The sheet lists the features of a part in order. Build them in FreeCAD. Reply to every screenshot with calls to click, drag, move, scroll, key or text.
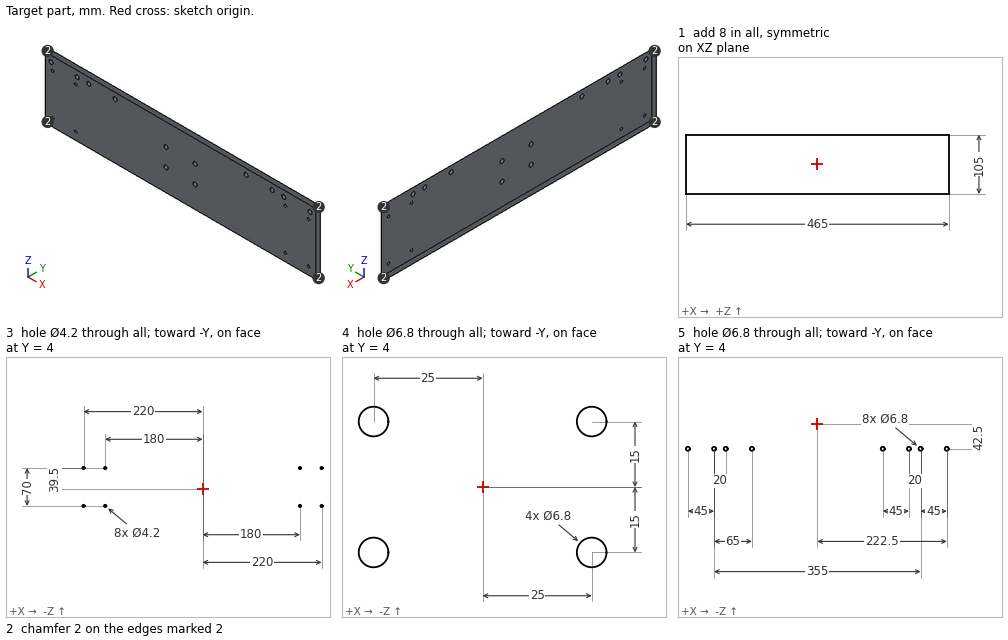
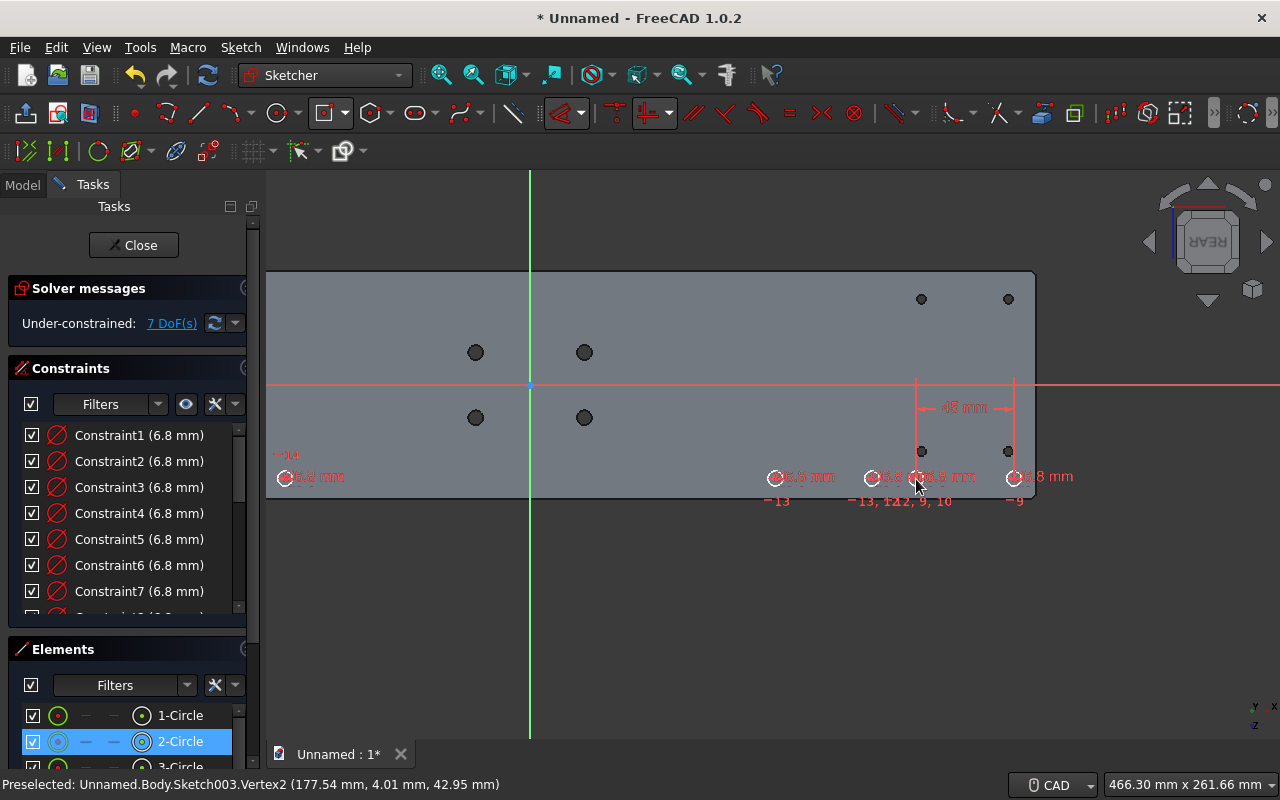
click(872, 479)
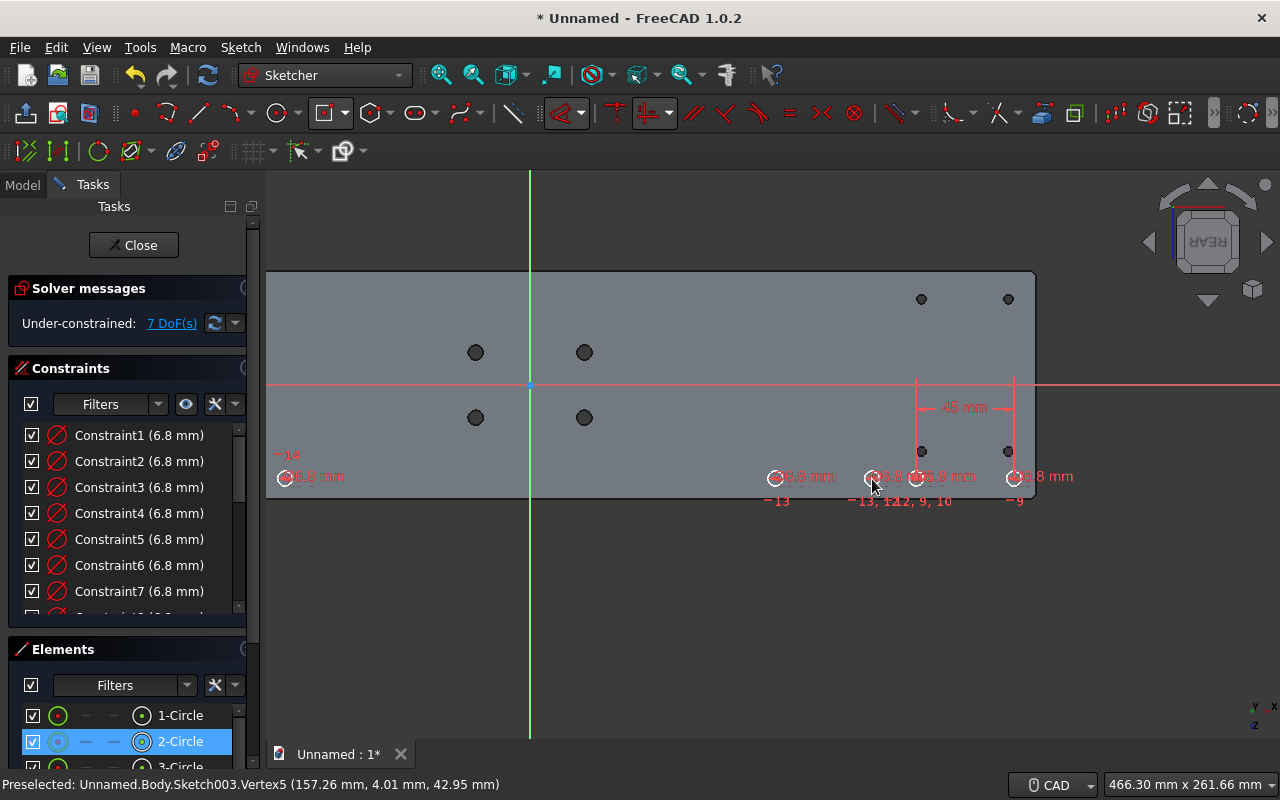
click(584, 114)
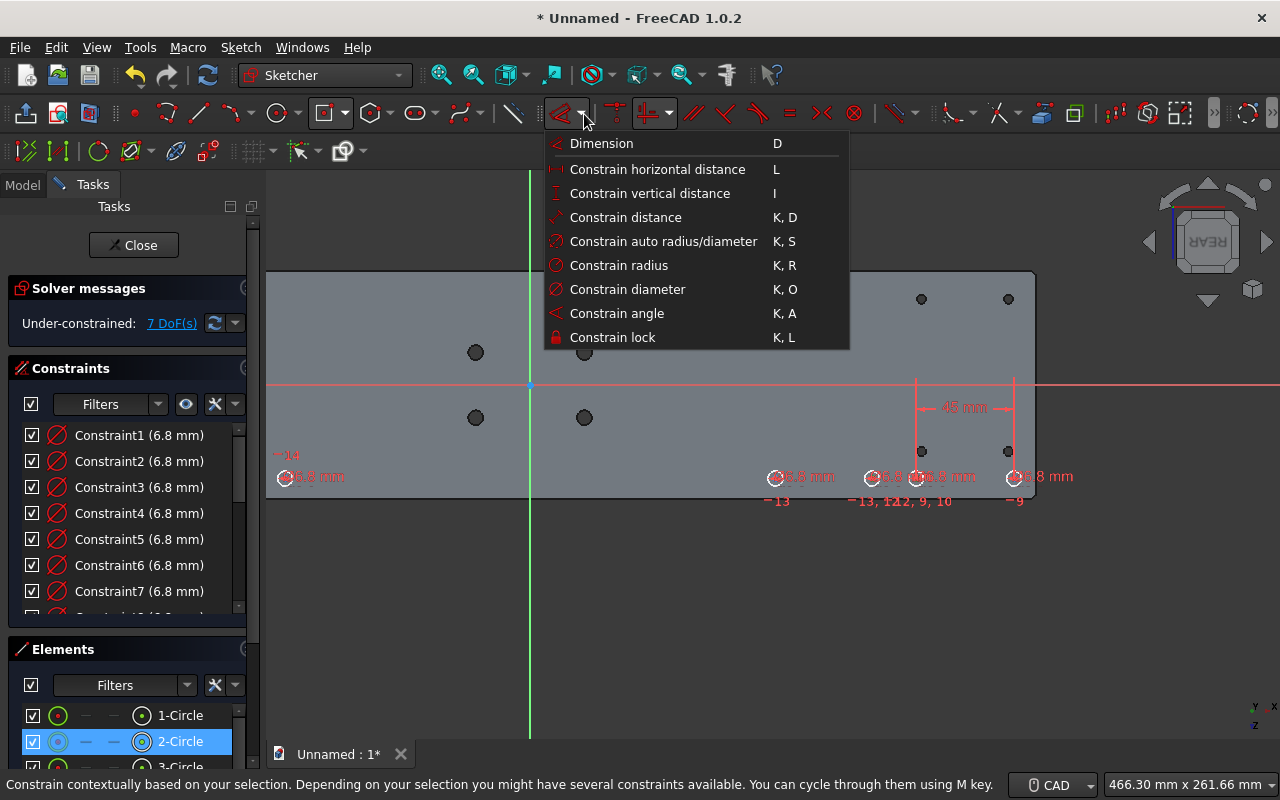
click(697, 169)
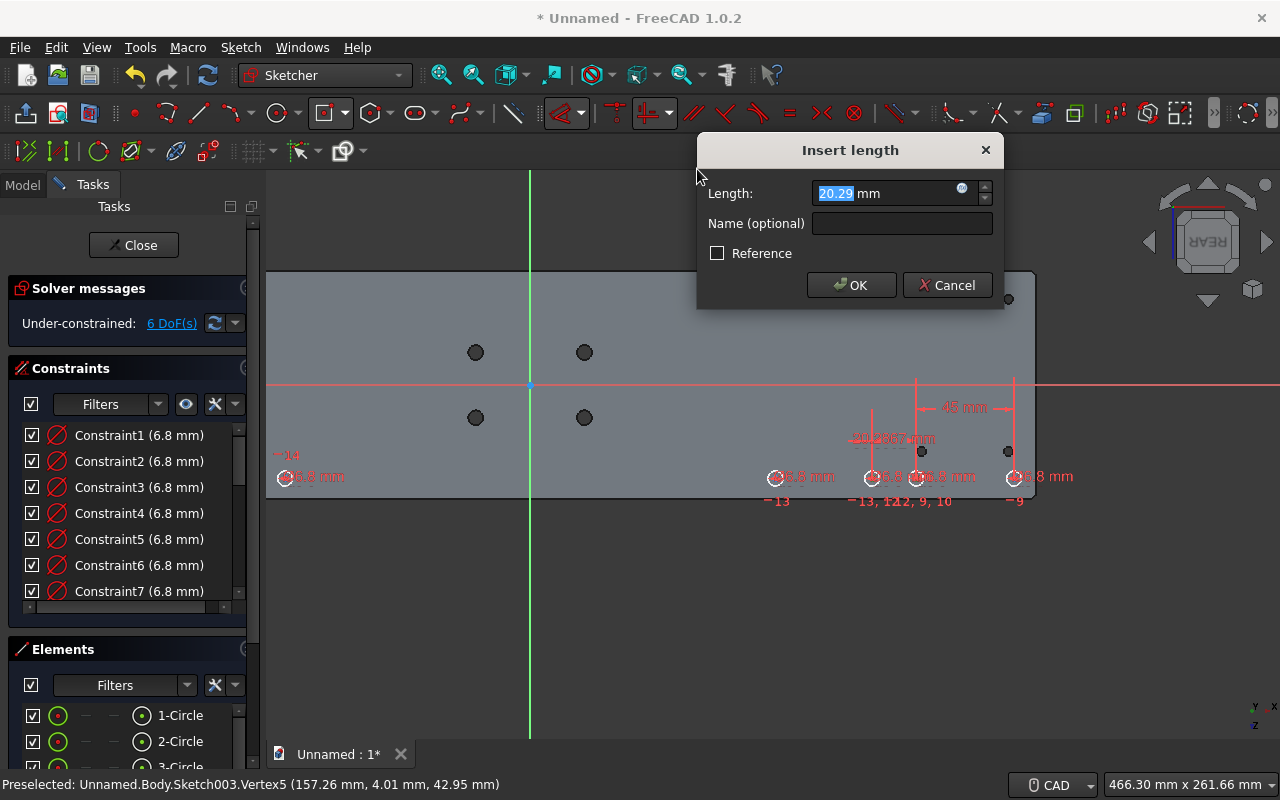
text(20)
key(Return)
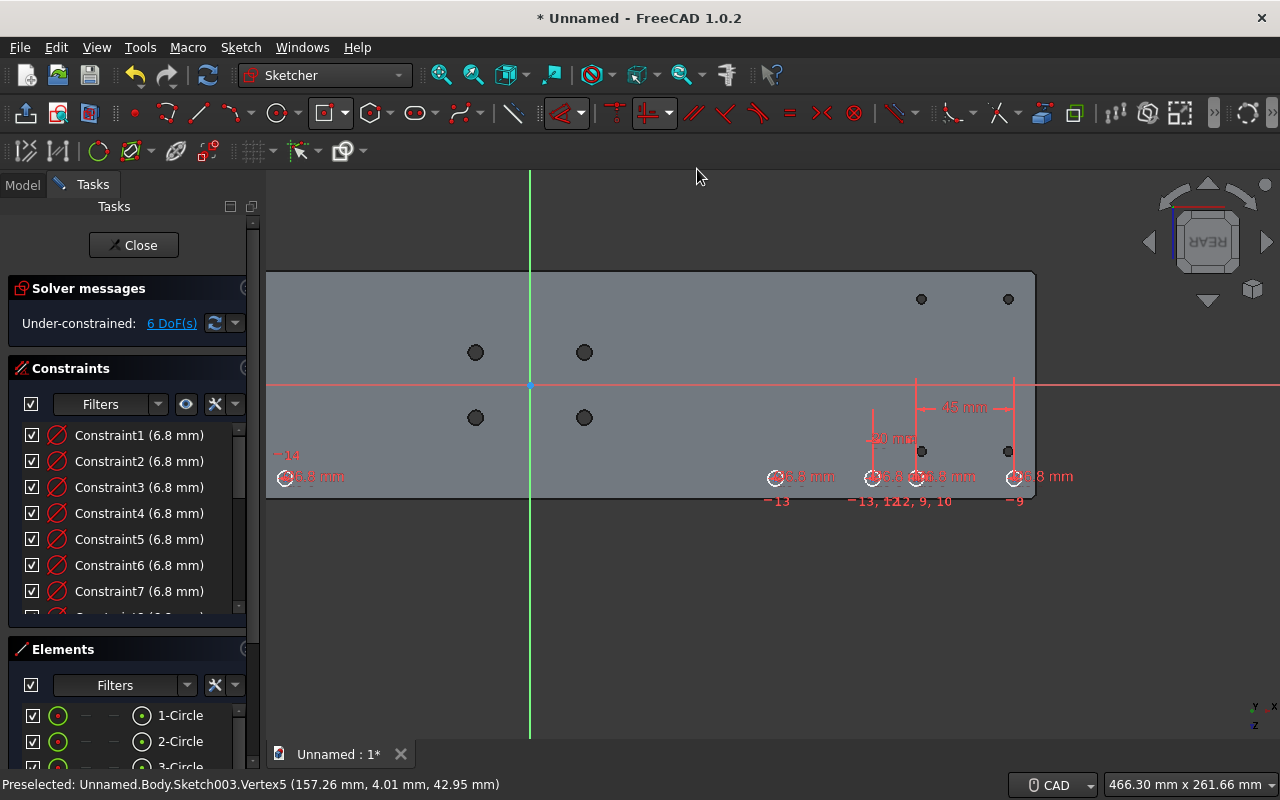
click(873, 479)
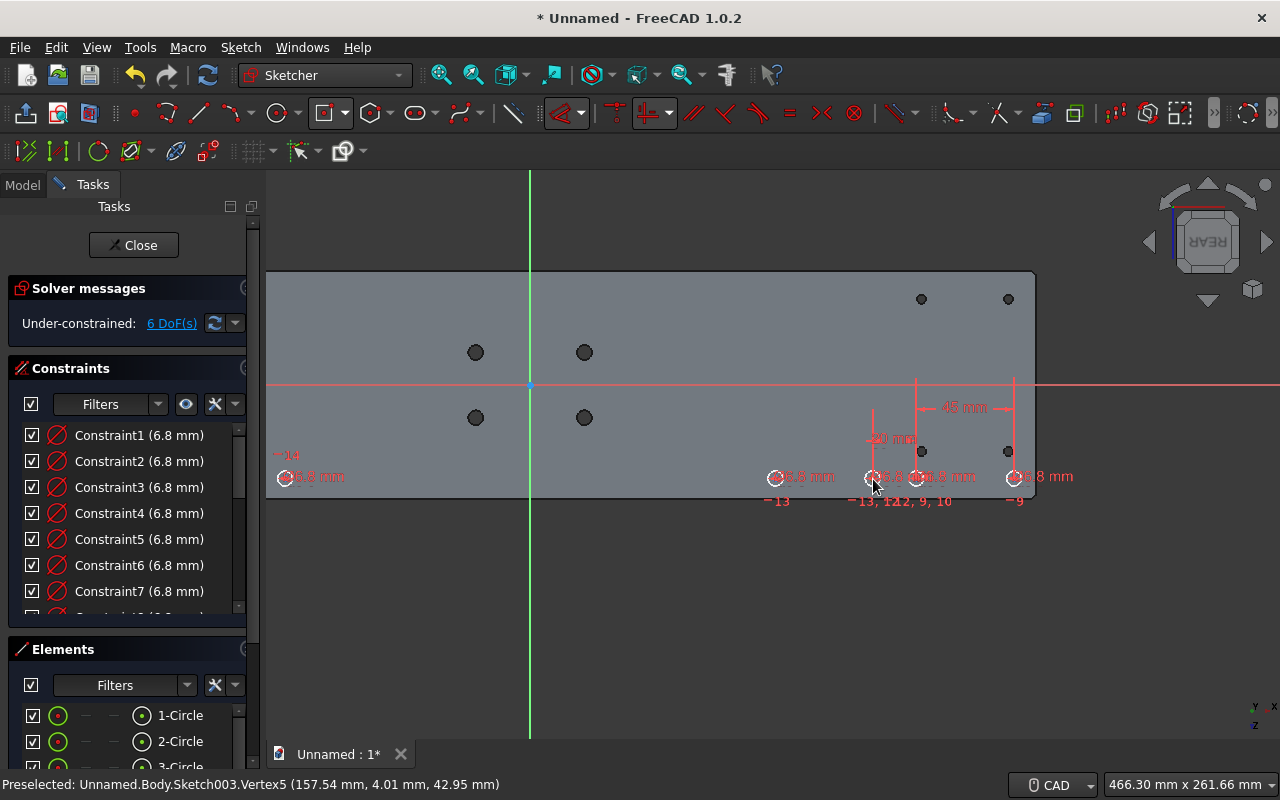
click(775, 479)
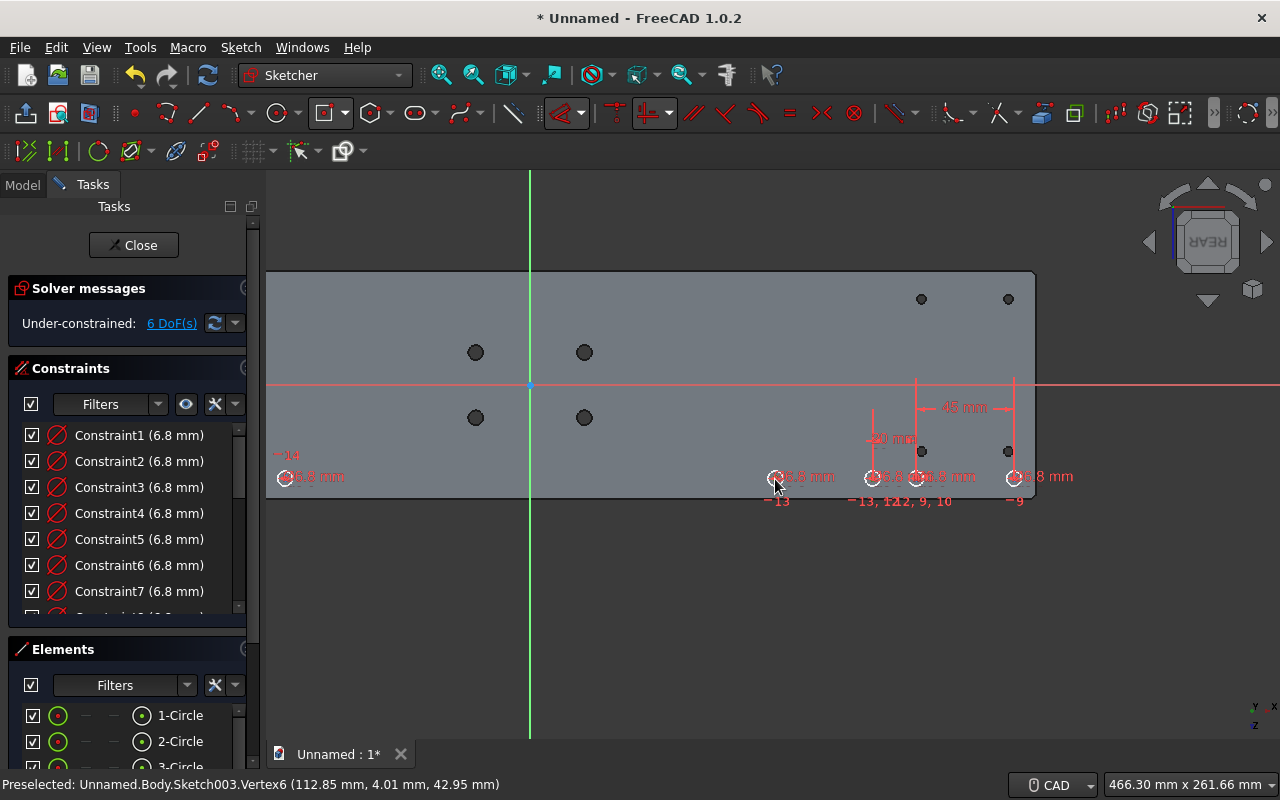
click(584, 114)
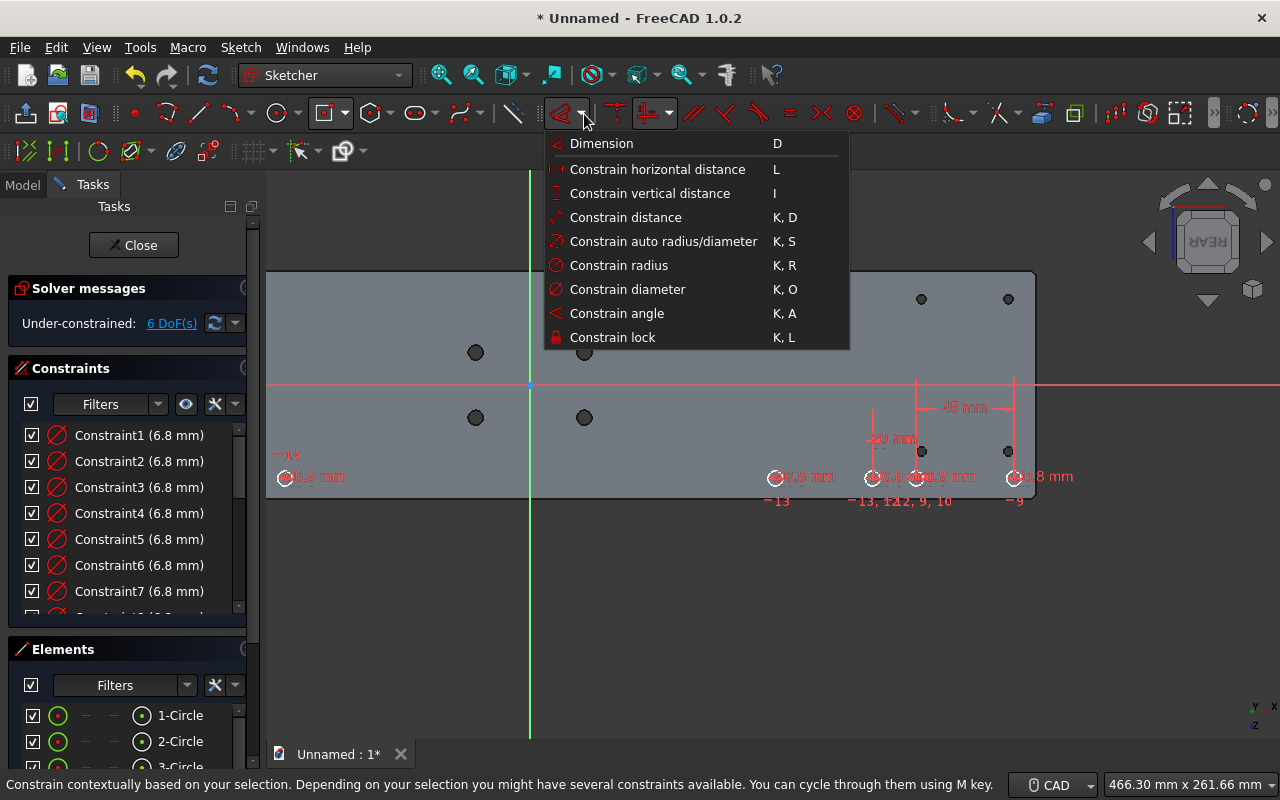
click(697, 169)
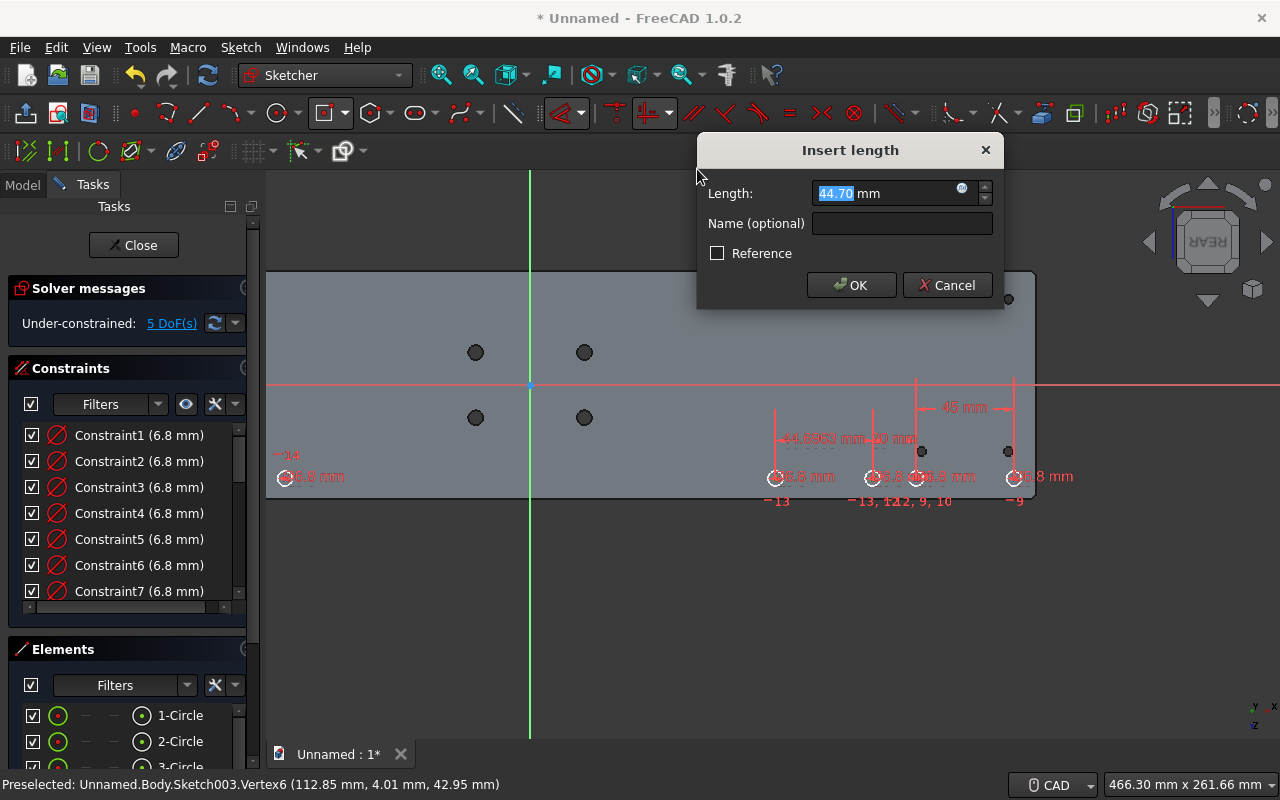
text(45)
key(Return)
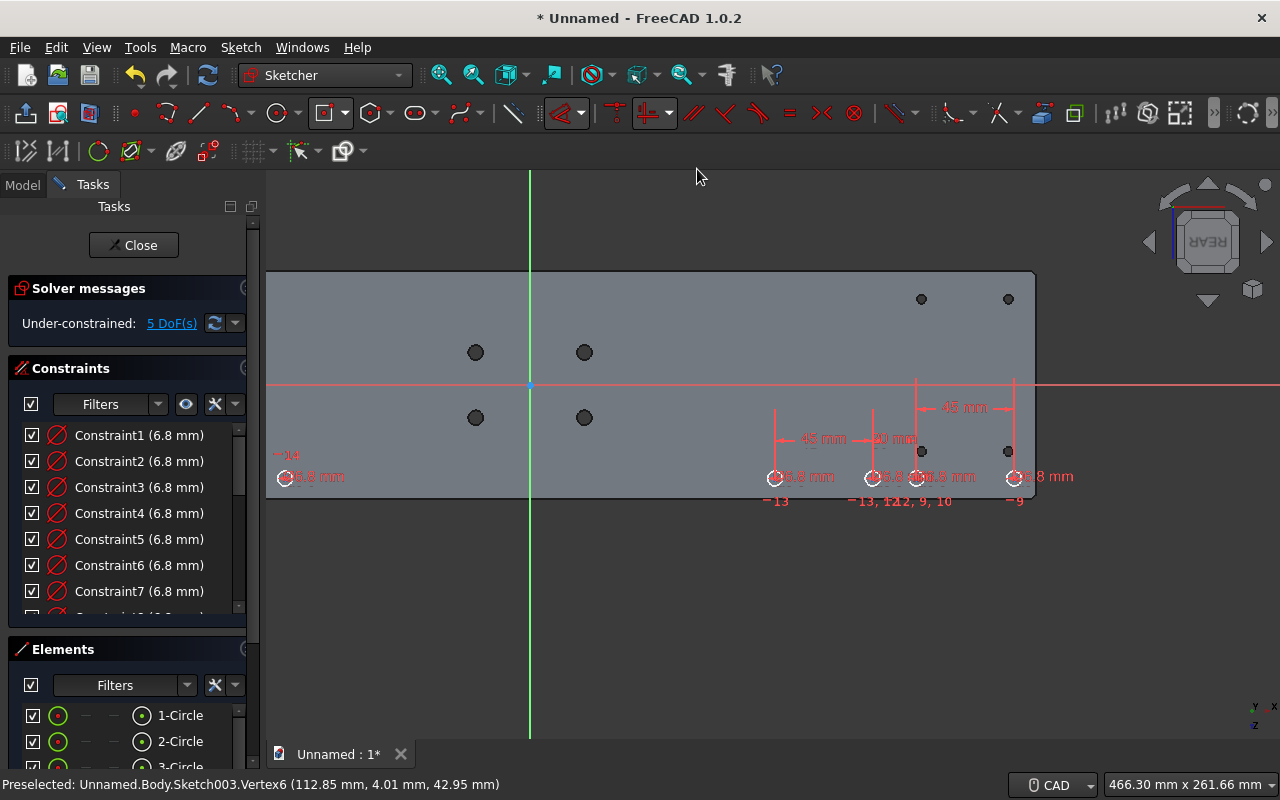
scroll(917, 478, down, 3)